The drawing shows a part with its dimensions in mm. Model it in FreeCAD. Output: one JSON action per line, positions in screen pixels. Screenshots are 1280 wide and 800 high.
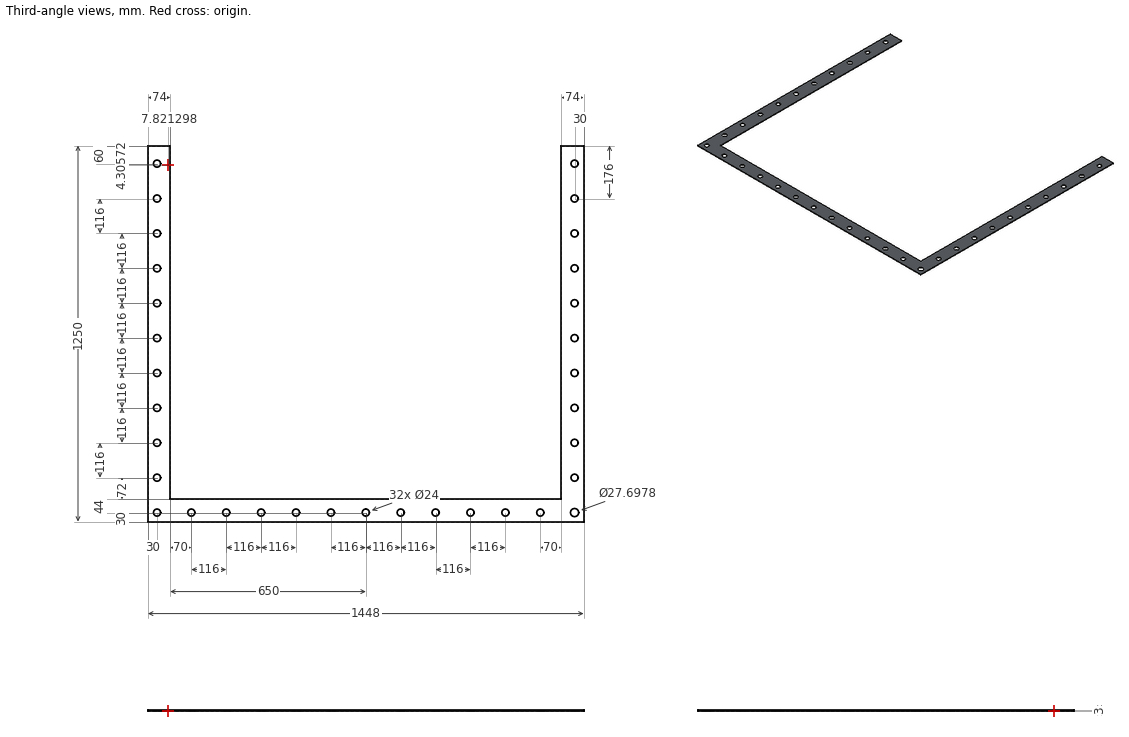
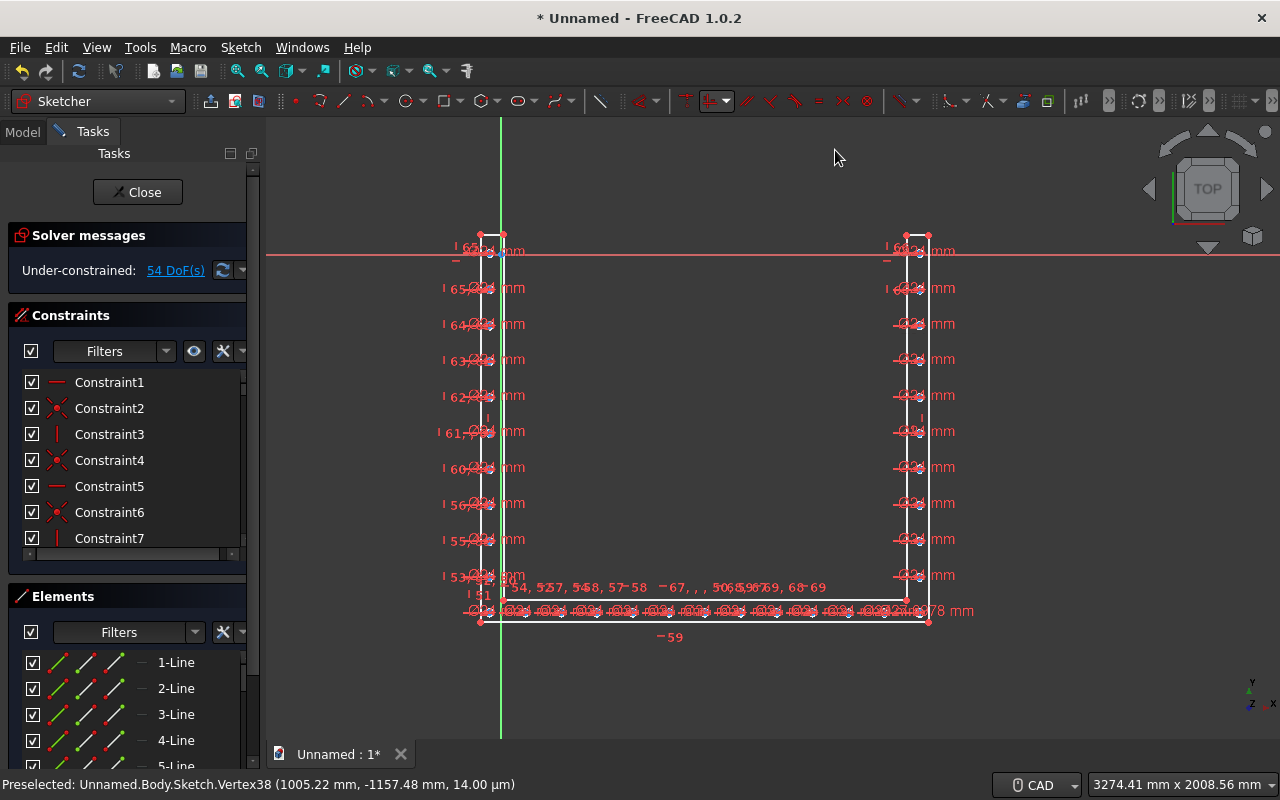
{"action": "left_click", "coordinate": [813, 613]}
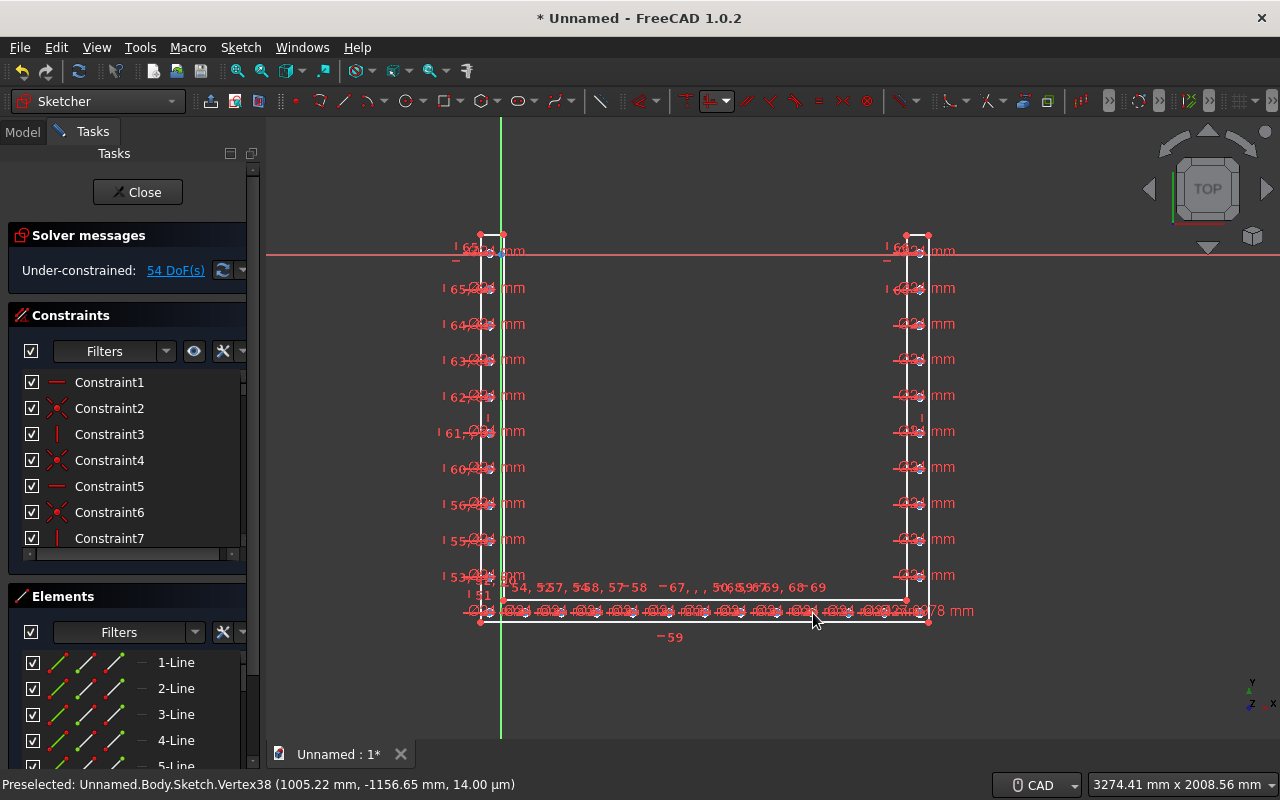
{"action": "left_click", "coordinate": [849, 613]}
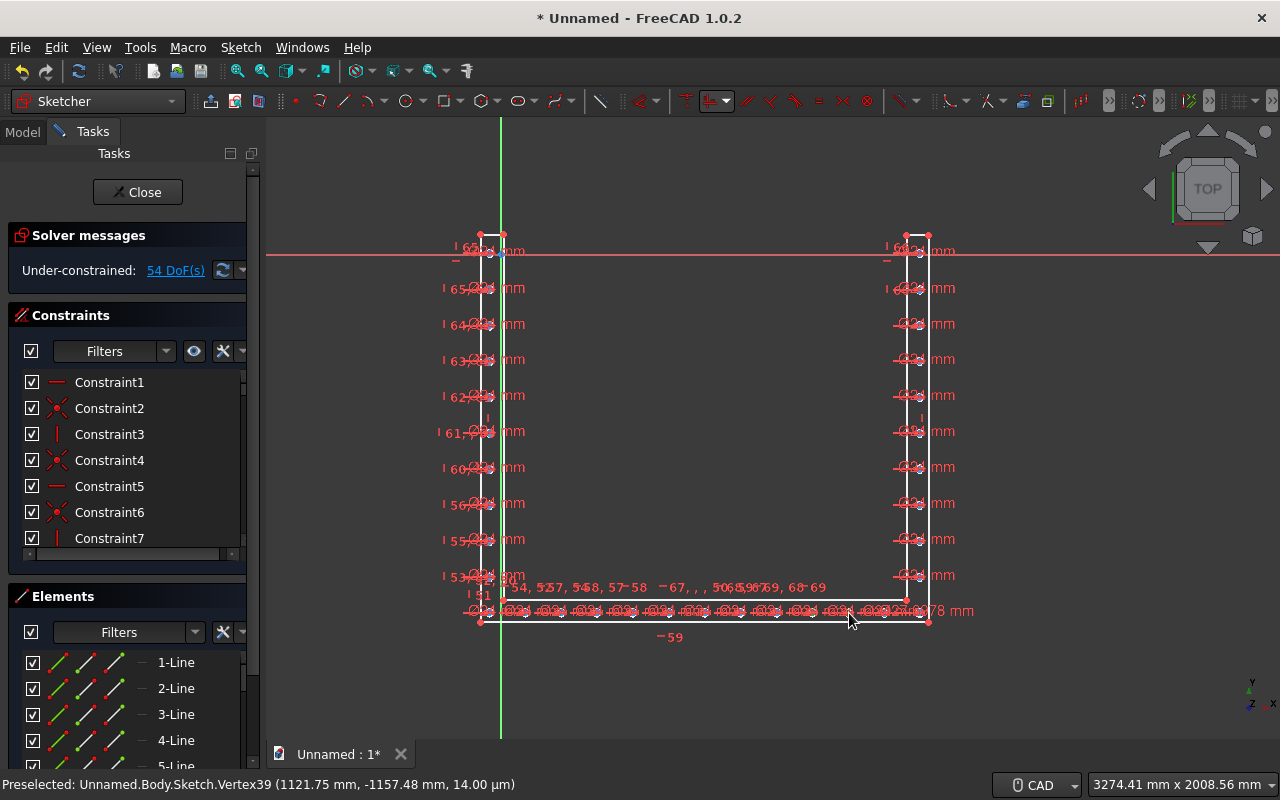
{"action": "key", "text": "h"}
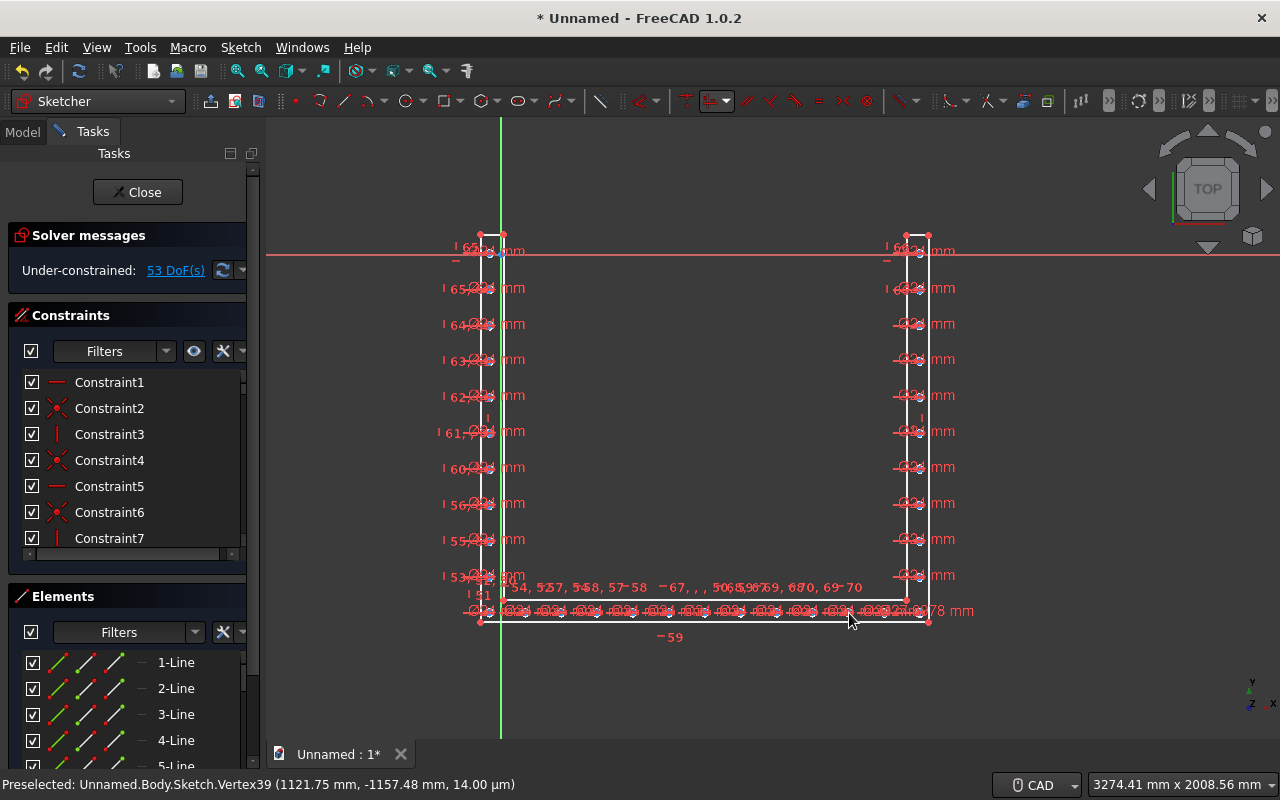
{"action": "left_click", "coordinate": [849, 613]}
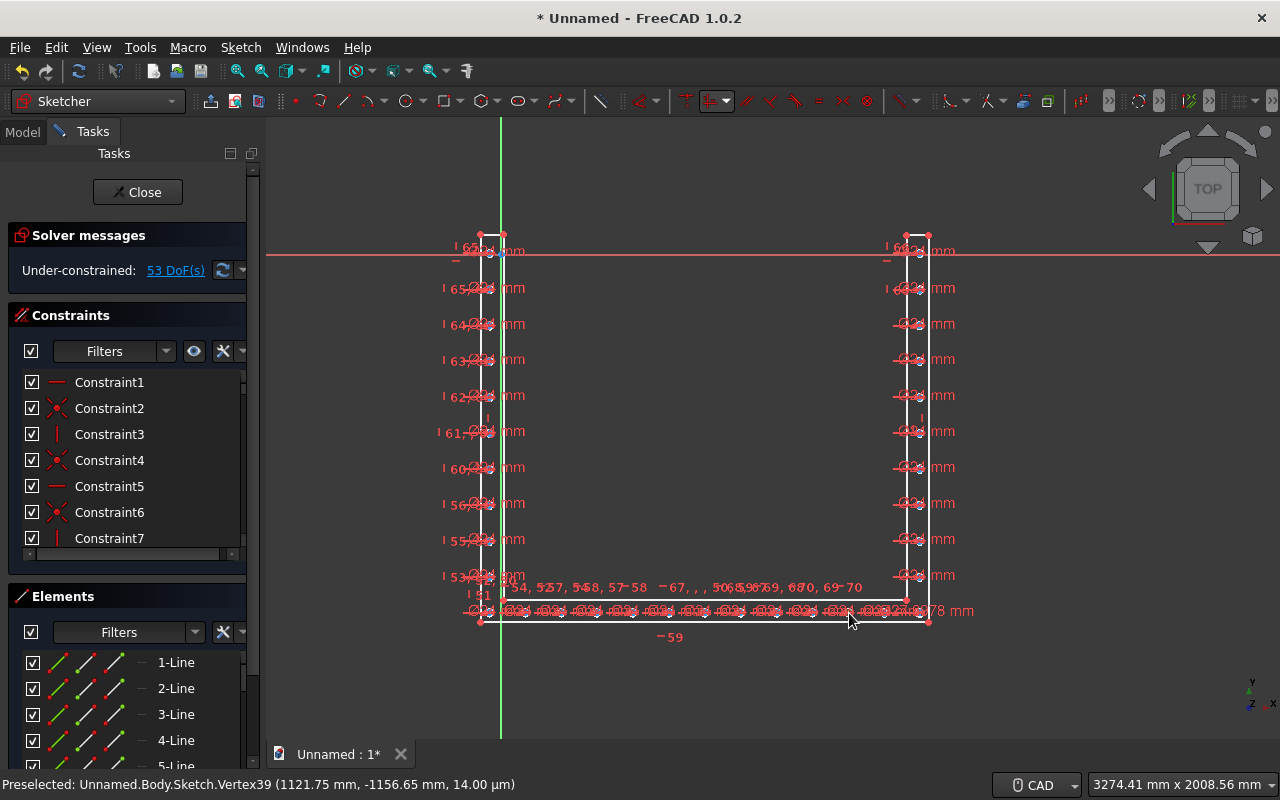
{"action": "left_click", "coordinate": [884, 613]}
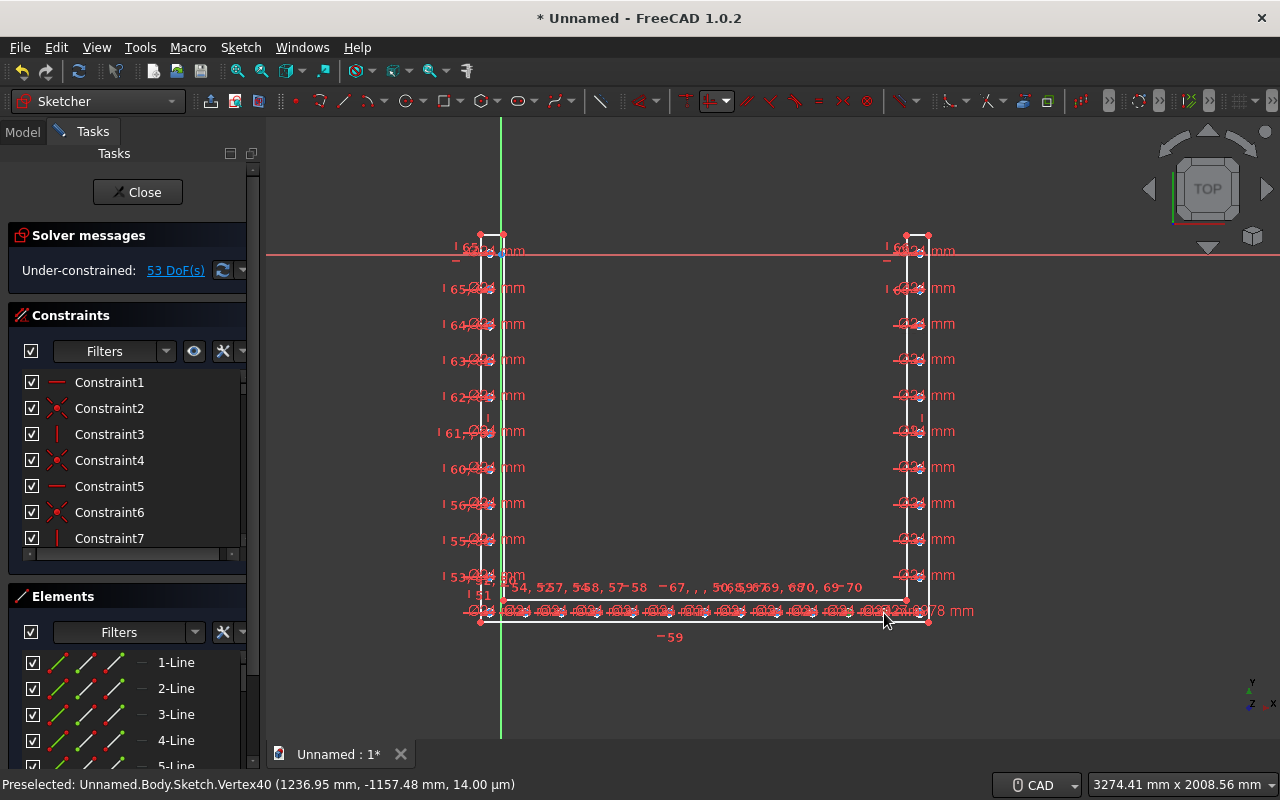
{"action": "key", "text": "h"}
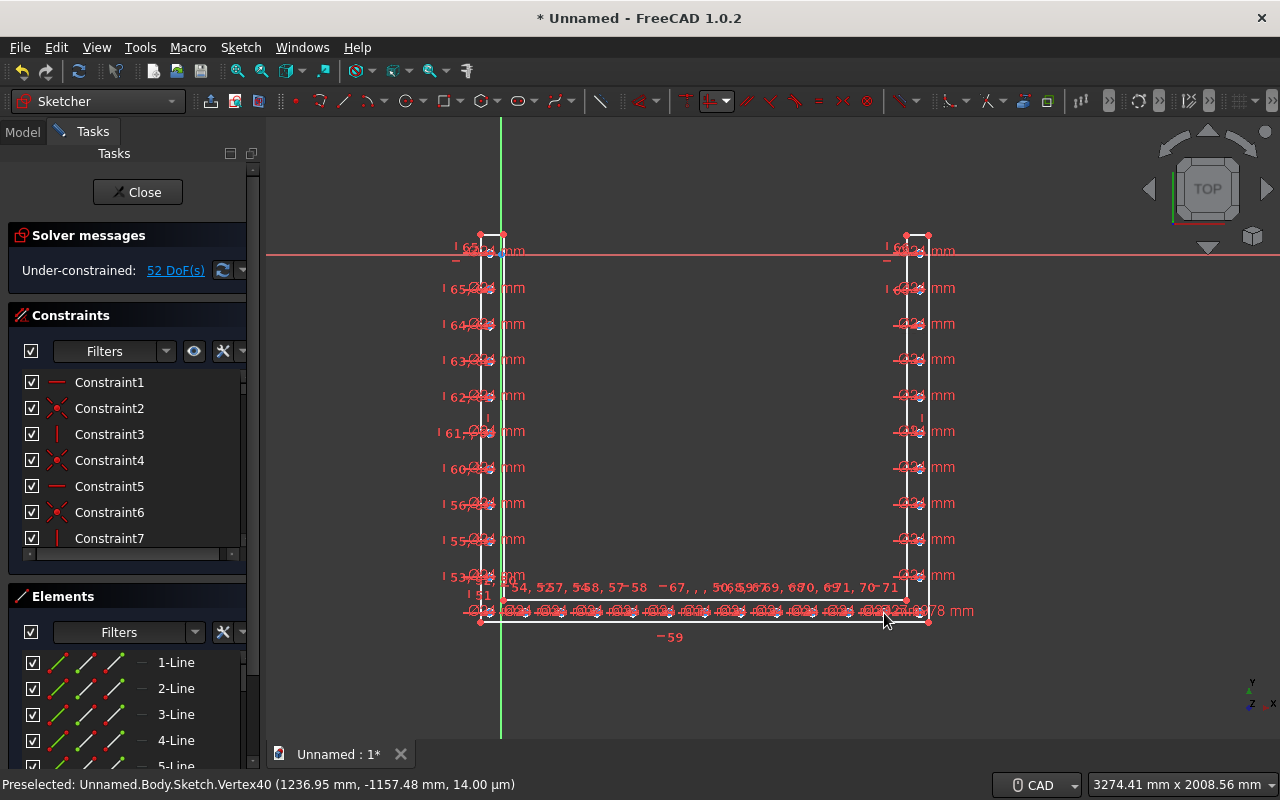
{"action": "left_click", "coordinate": [884, 613]}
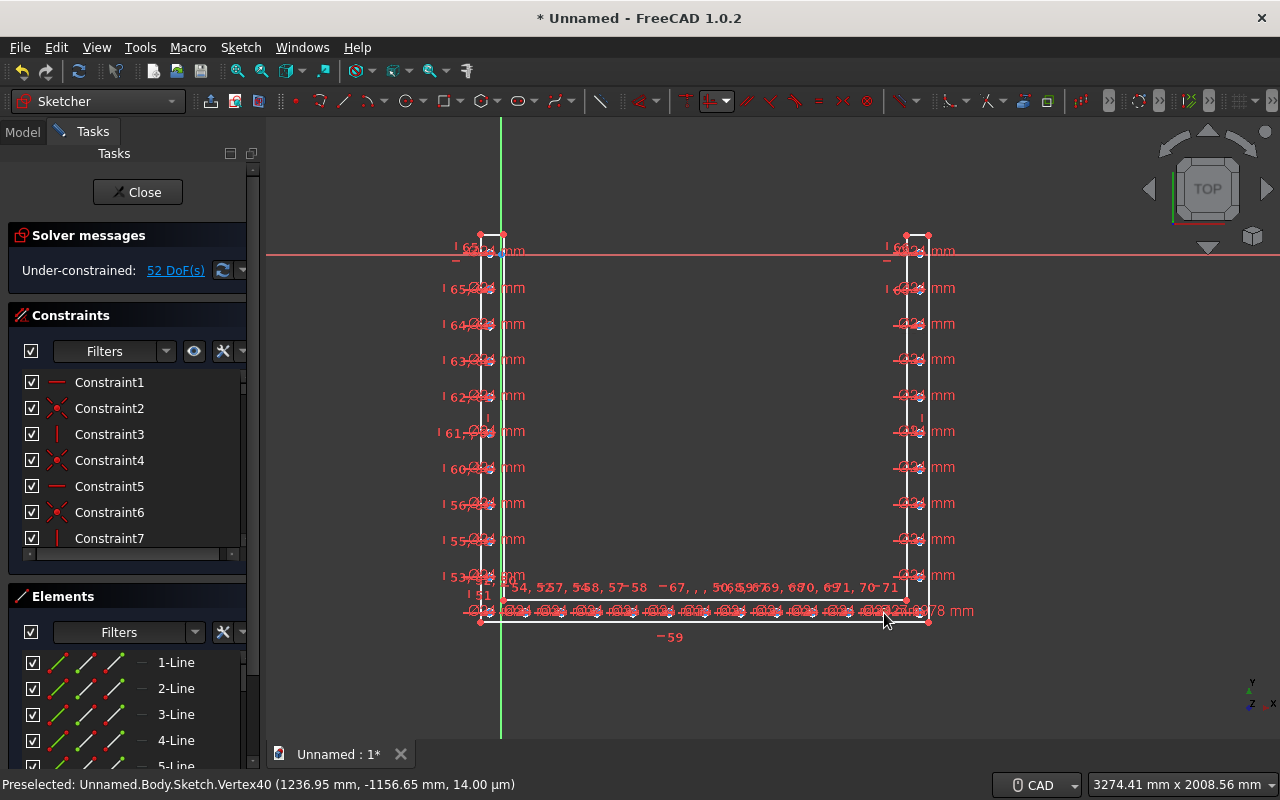
{"action": "left_click", "coordinate": [920, 613]}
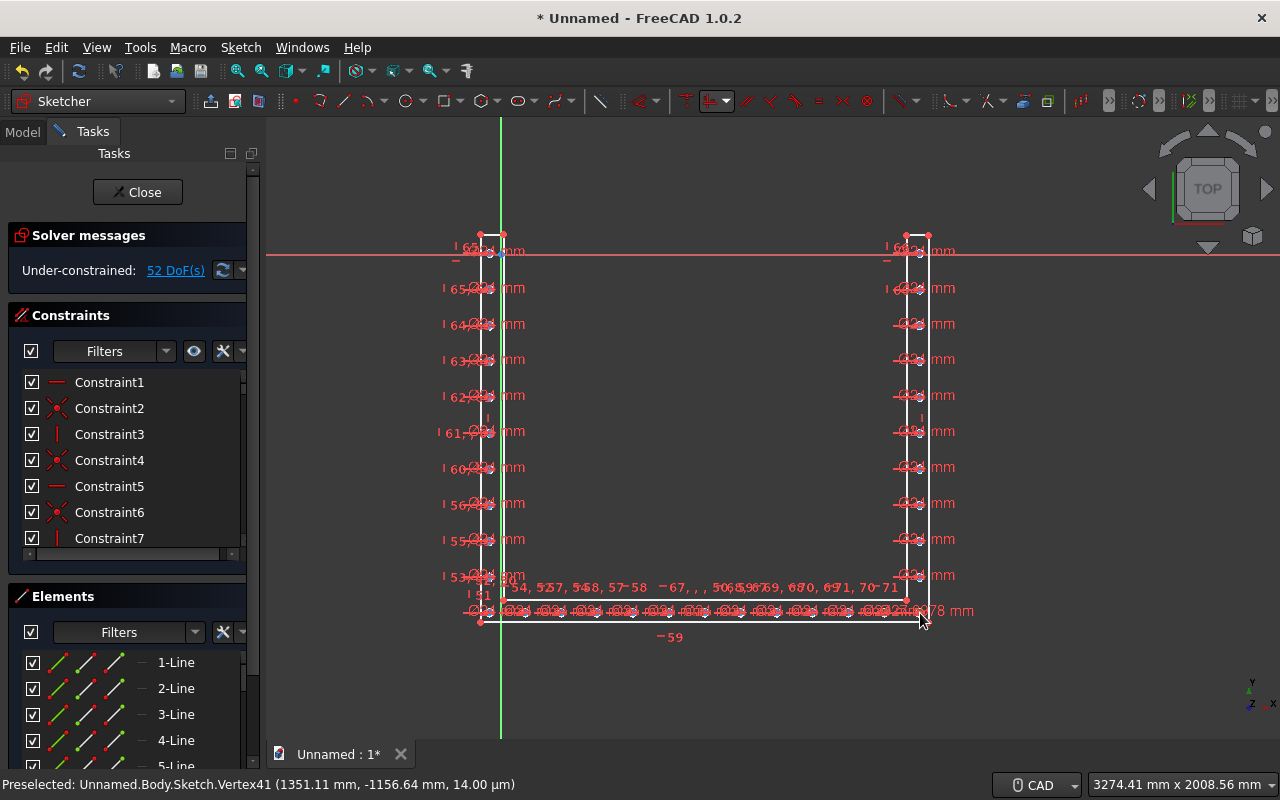
{"action": "key", "text": "h"}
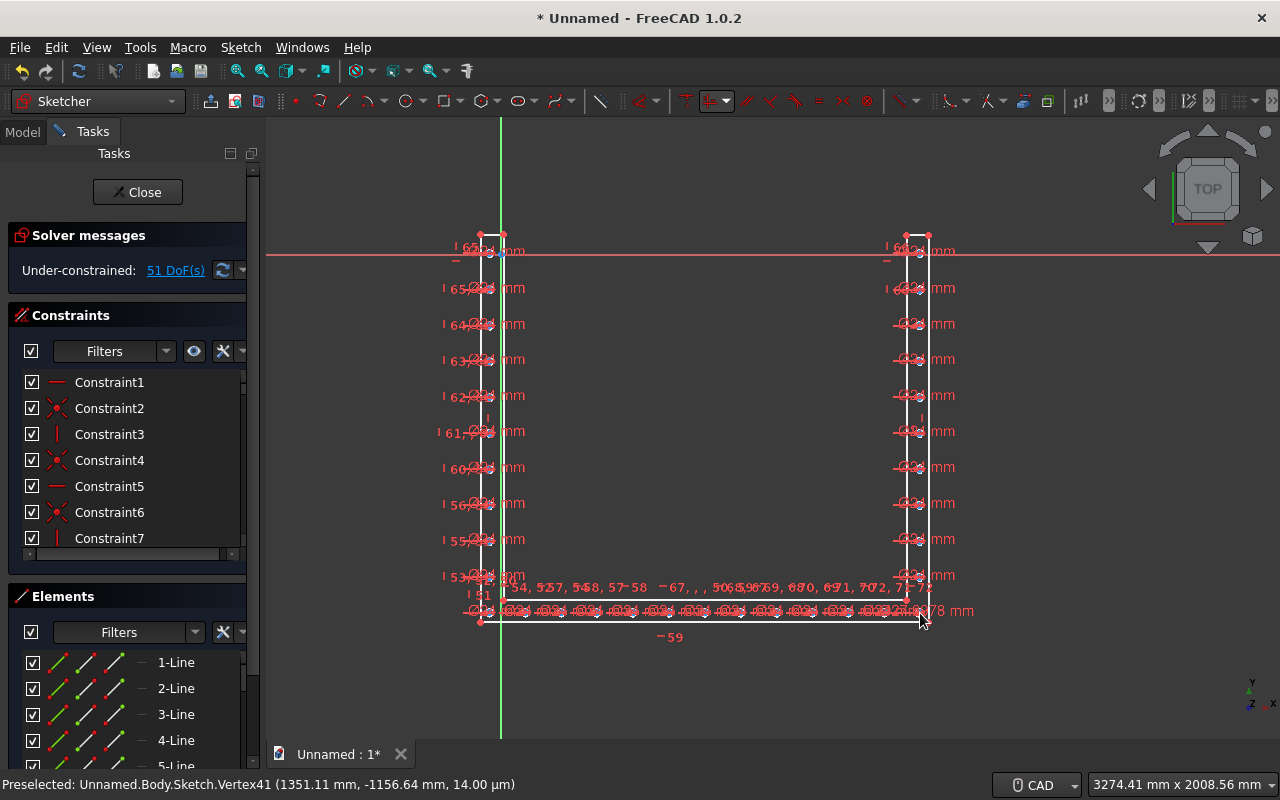
{"action": "left_click", "coordinate": [920, 613]}